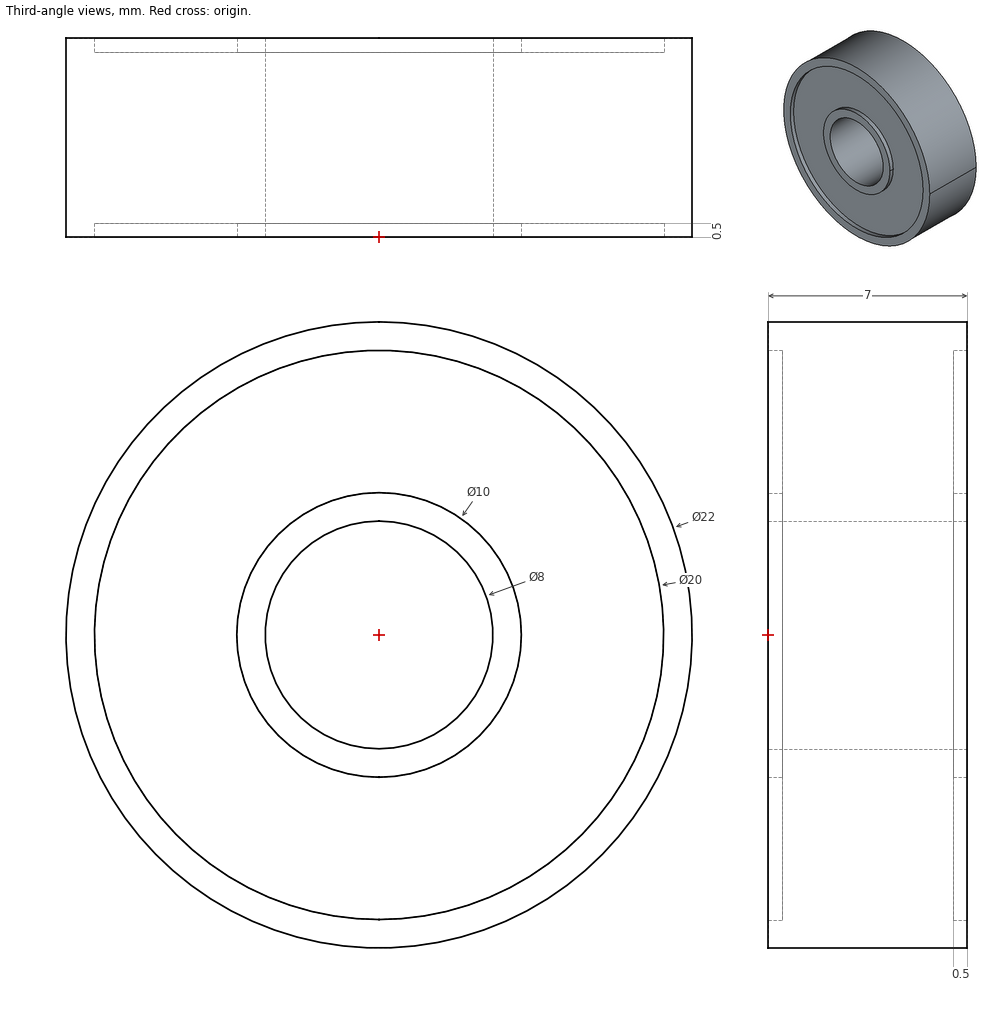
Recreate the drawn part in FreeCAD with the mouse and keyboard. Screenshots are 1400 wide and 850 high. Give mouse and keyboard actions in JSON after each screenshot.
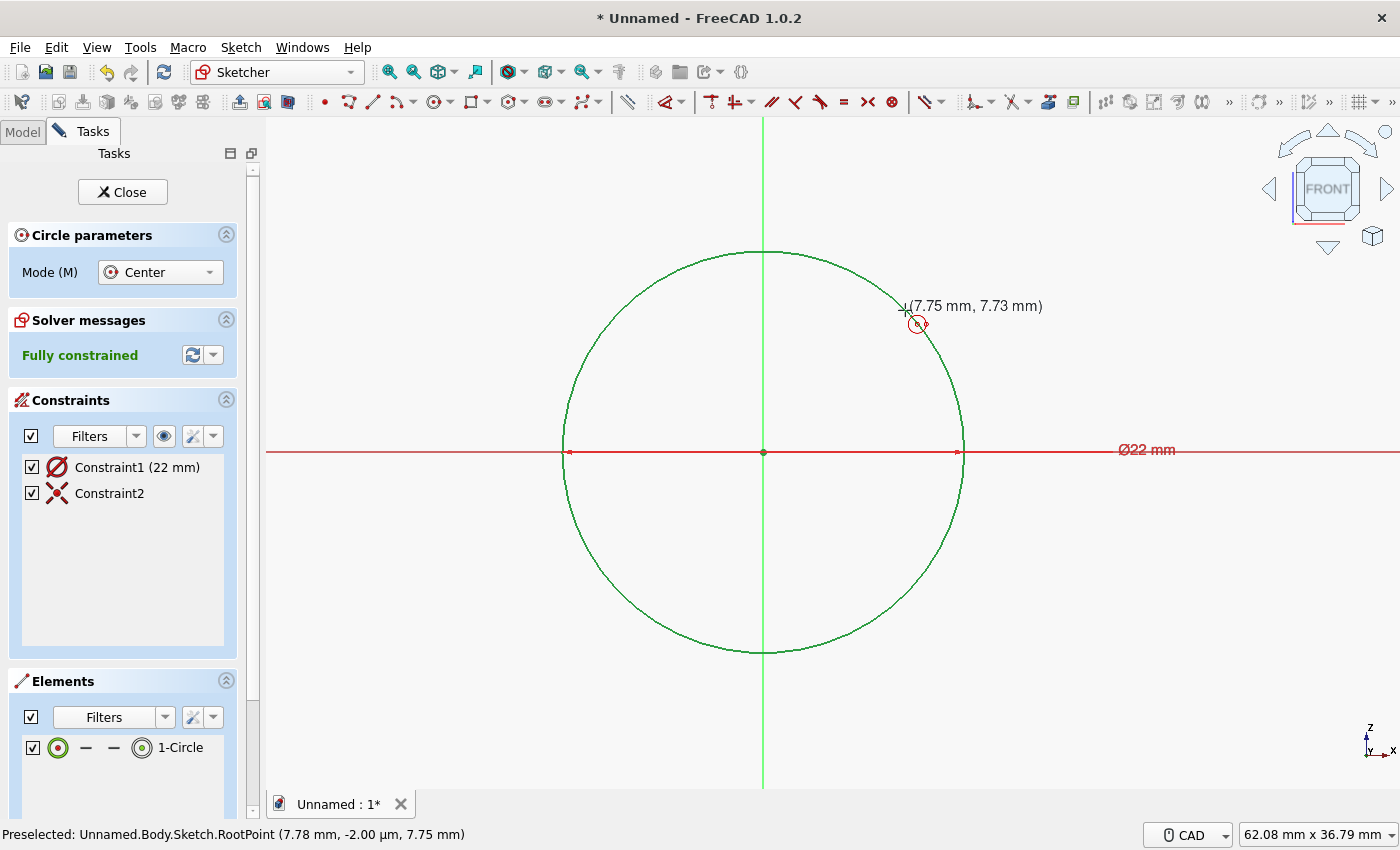
{"action": "left_click", "coordinate": [763, 452]}
{"action": "mouse_move", "coordinate": [815, 400]}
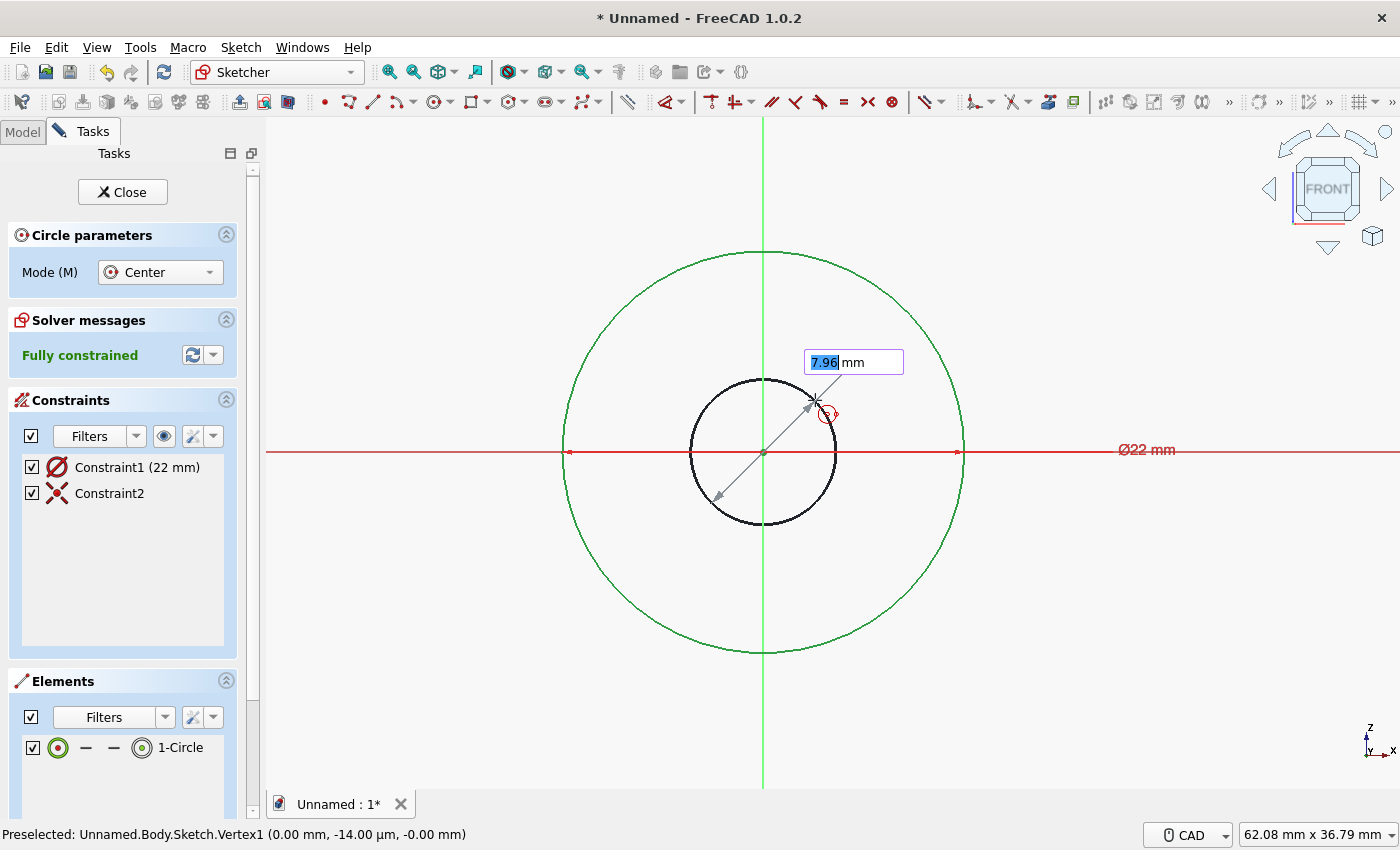
{"action": "type", "text": "8"}
{"action": "key", "text": "Return"}
{"action": "key", "text": "Escape"}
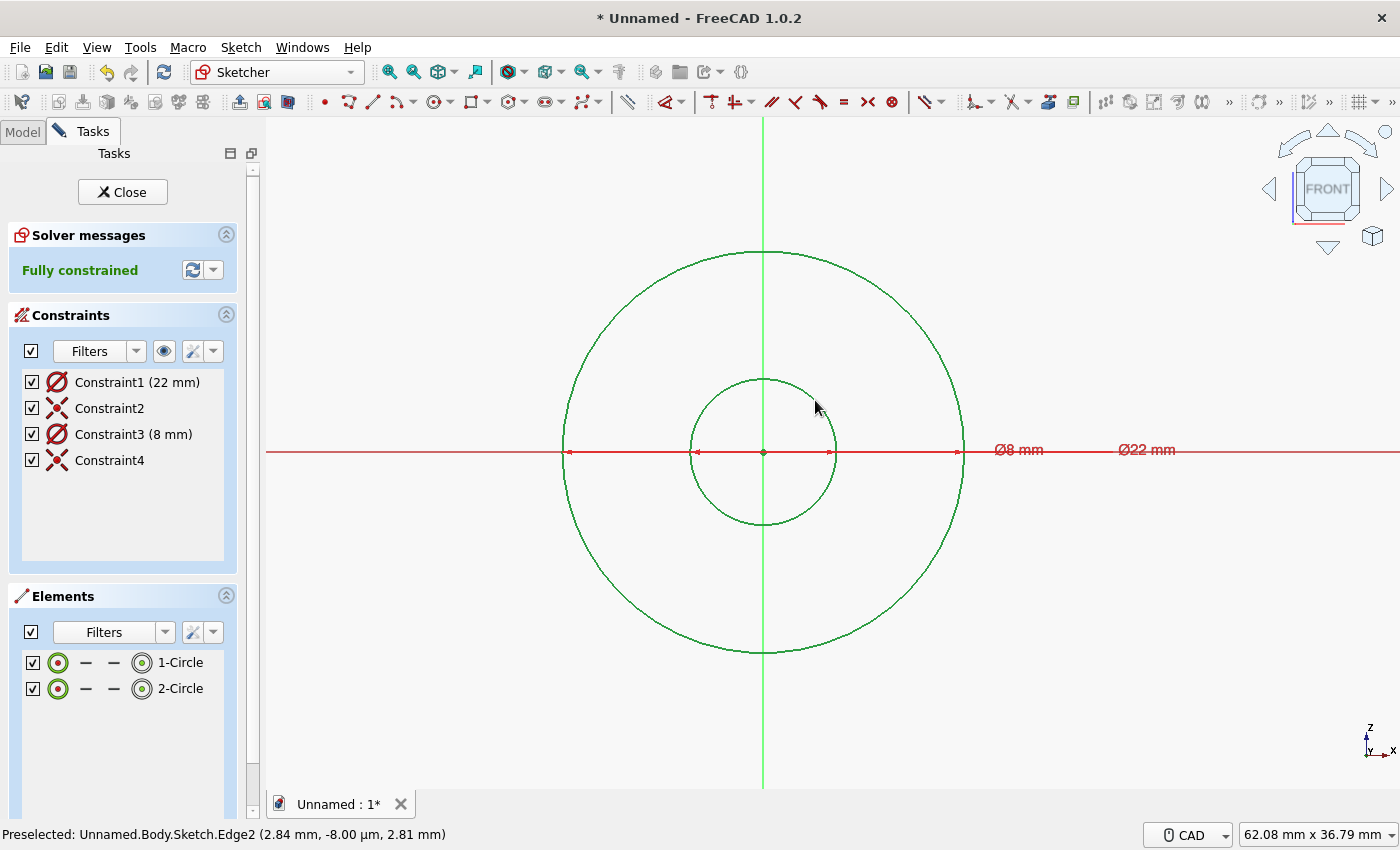
{"action": "left_click", "coordinate": [123, 192]}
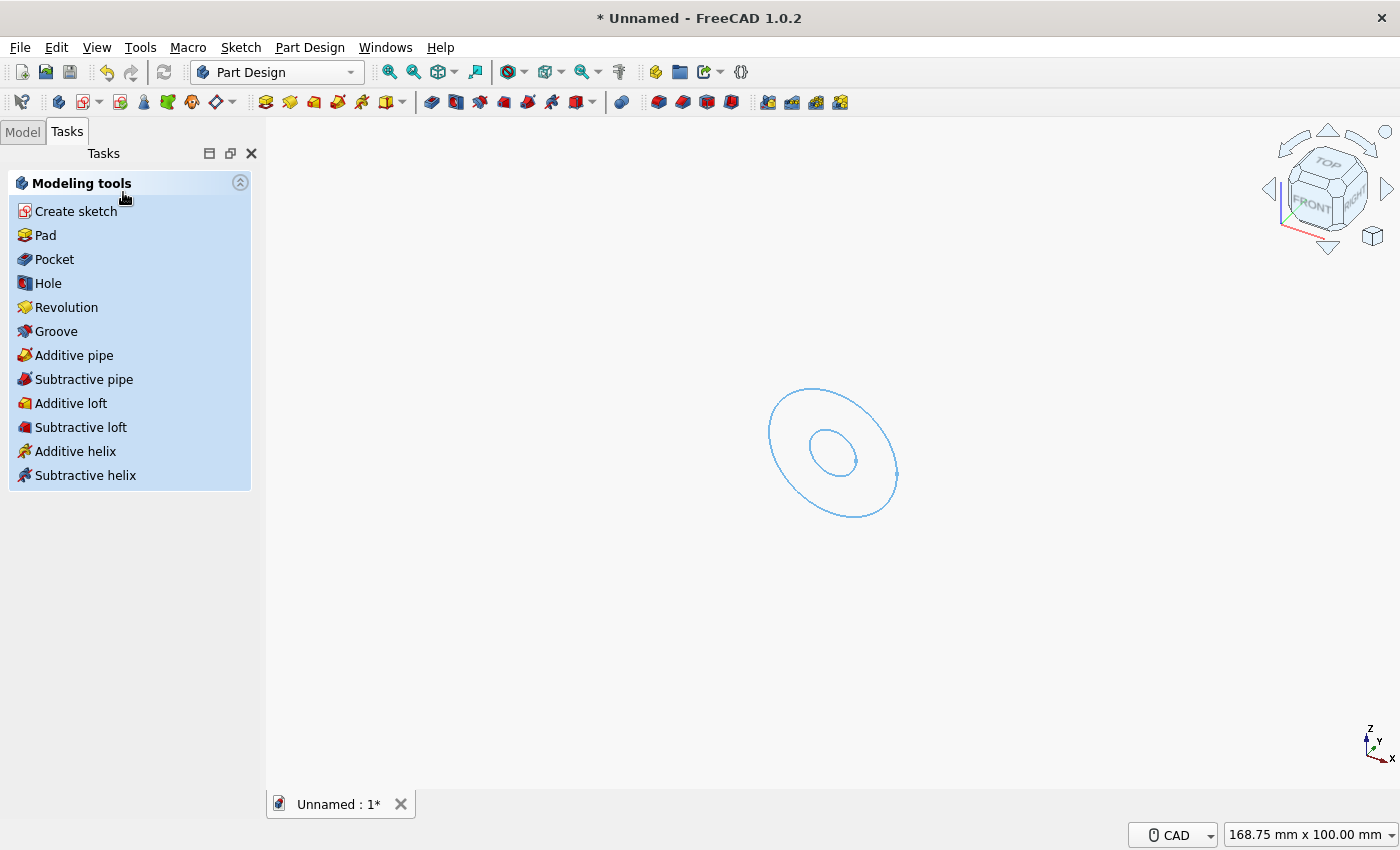
{"action": "left_click", "coordinate": [266, 102]}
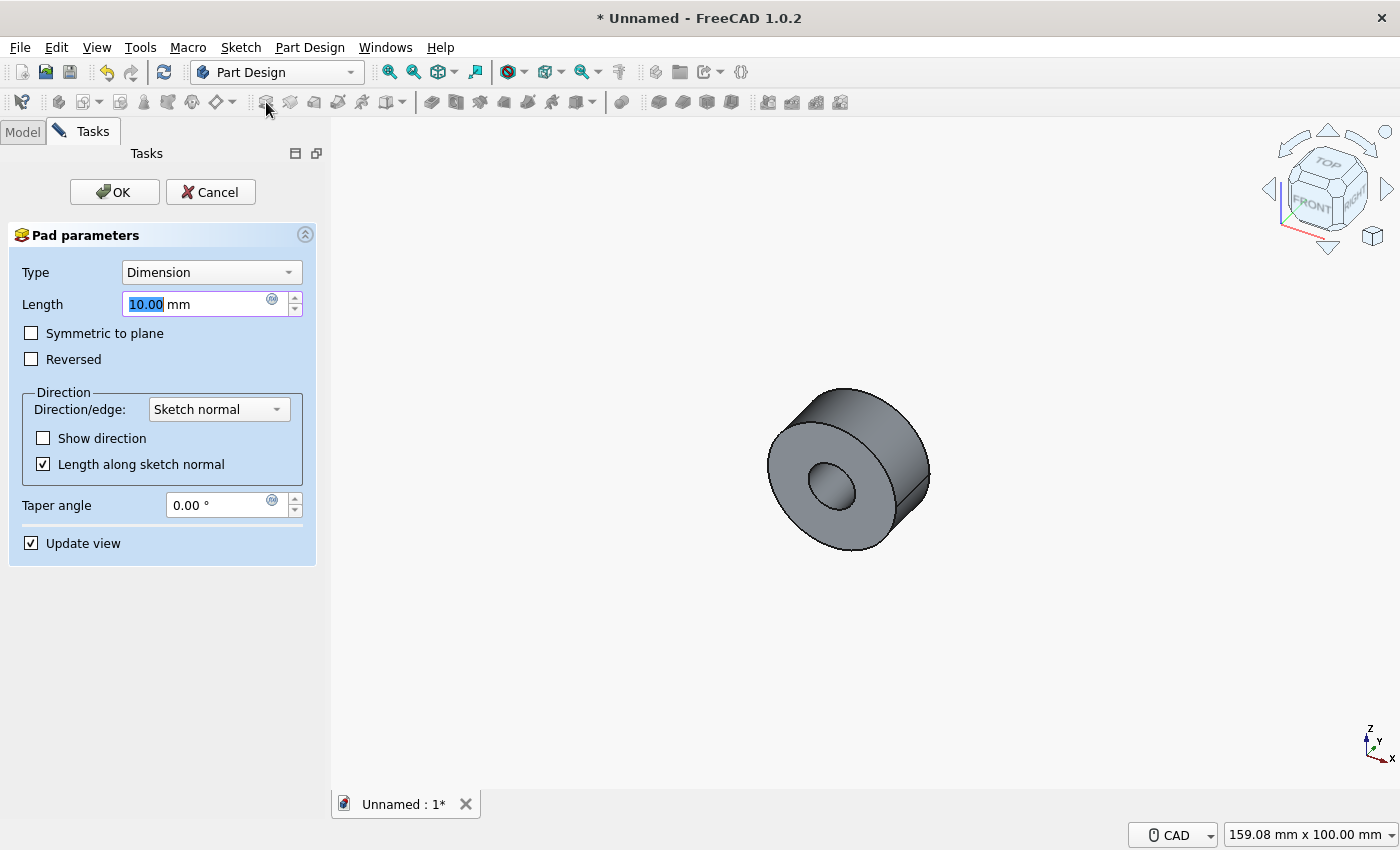
{"action": "type", "text": "7"}
{"action": "key", "text": "Tab"}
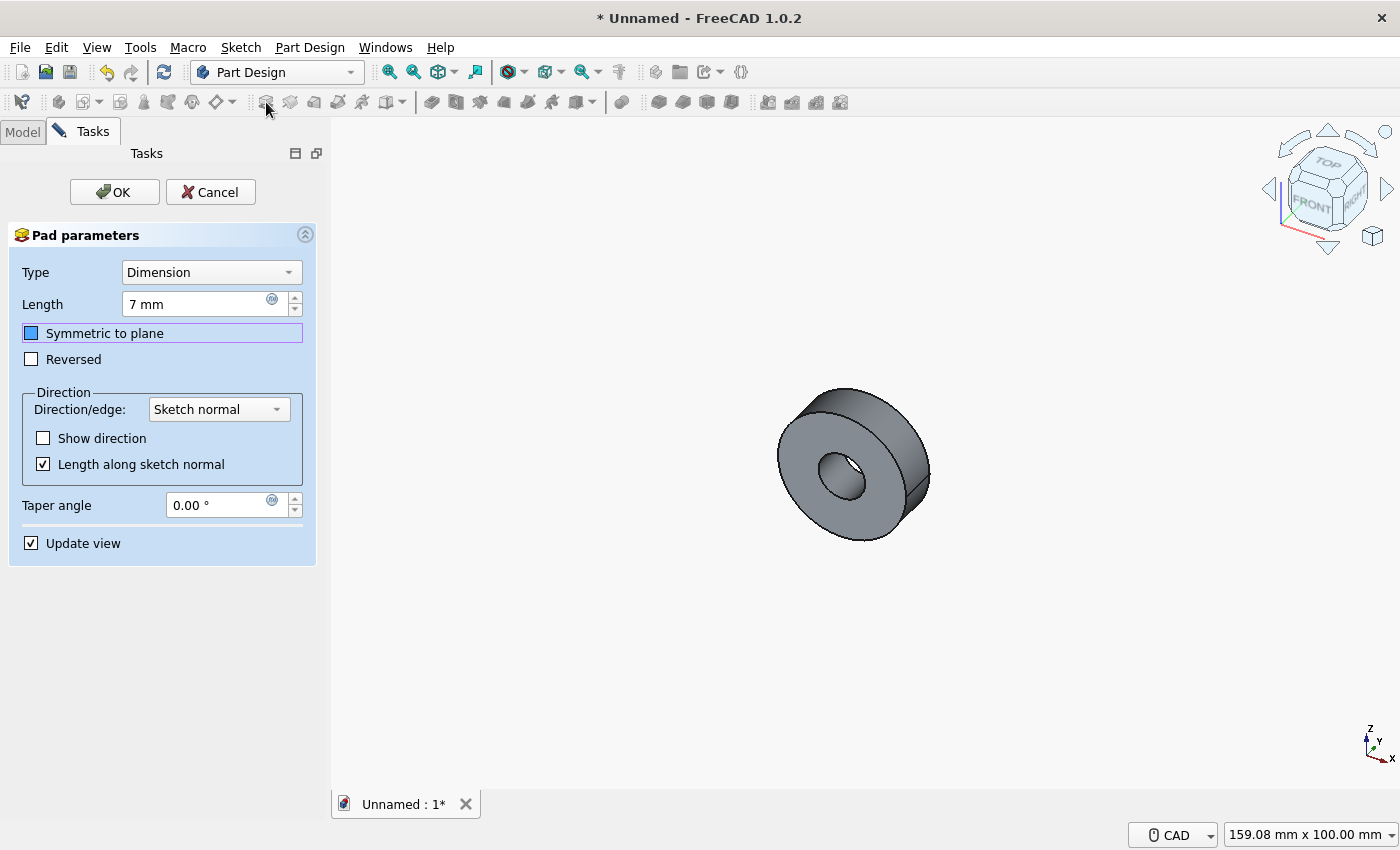
{"action": "left_click", "coordinate": [30, 359]}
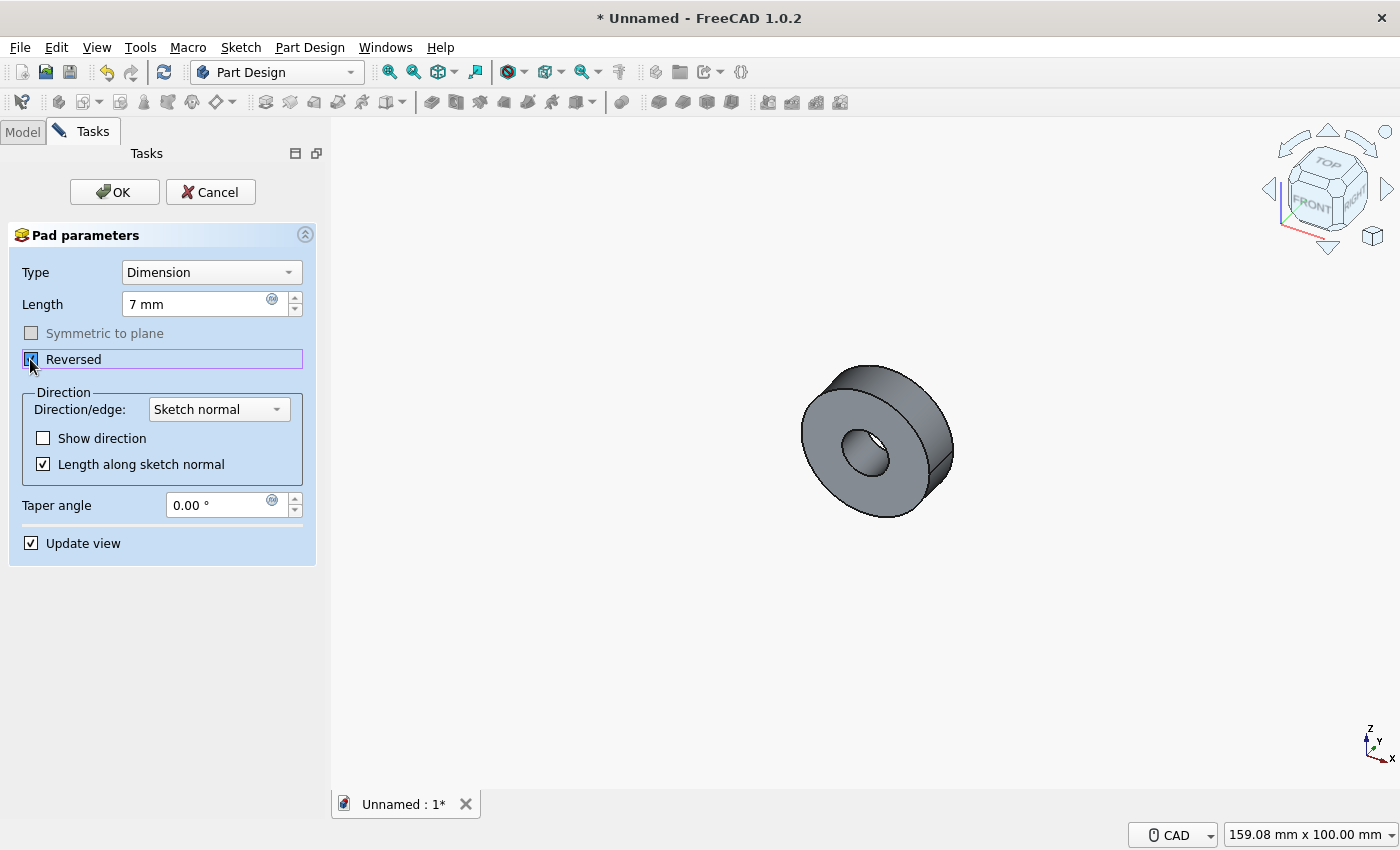
{"action": "left_click", "coordinate": [115, 192]}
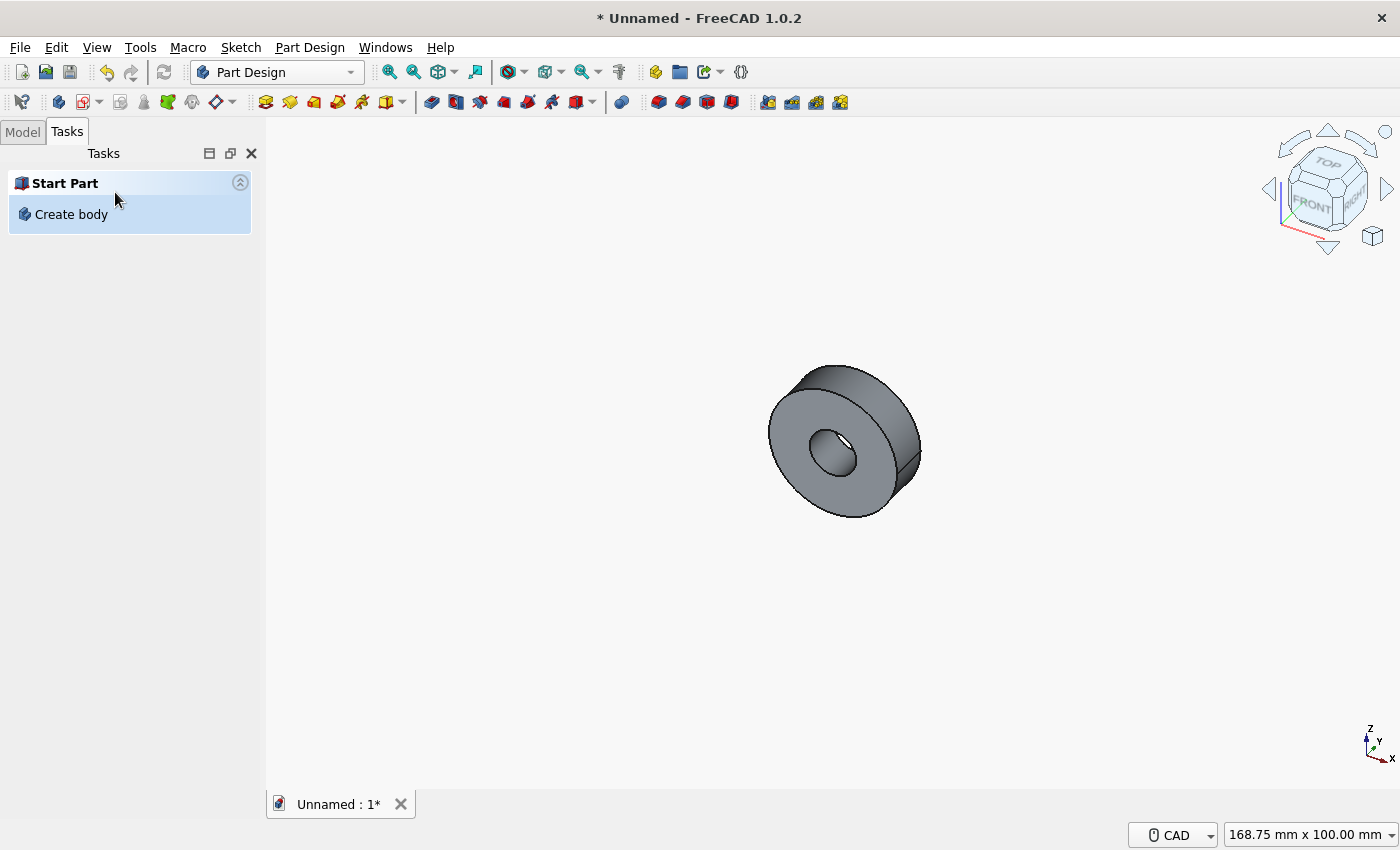
{"action": "key", "text": "v f"}